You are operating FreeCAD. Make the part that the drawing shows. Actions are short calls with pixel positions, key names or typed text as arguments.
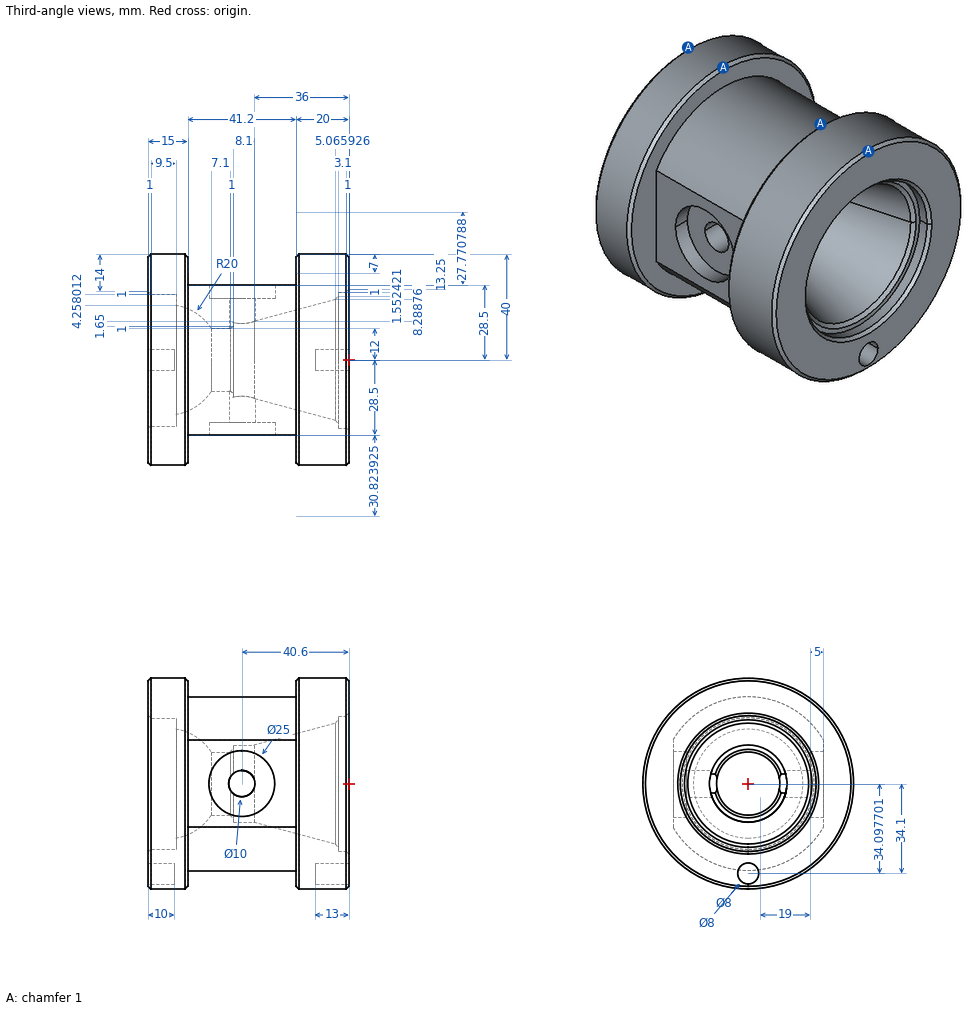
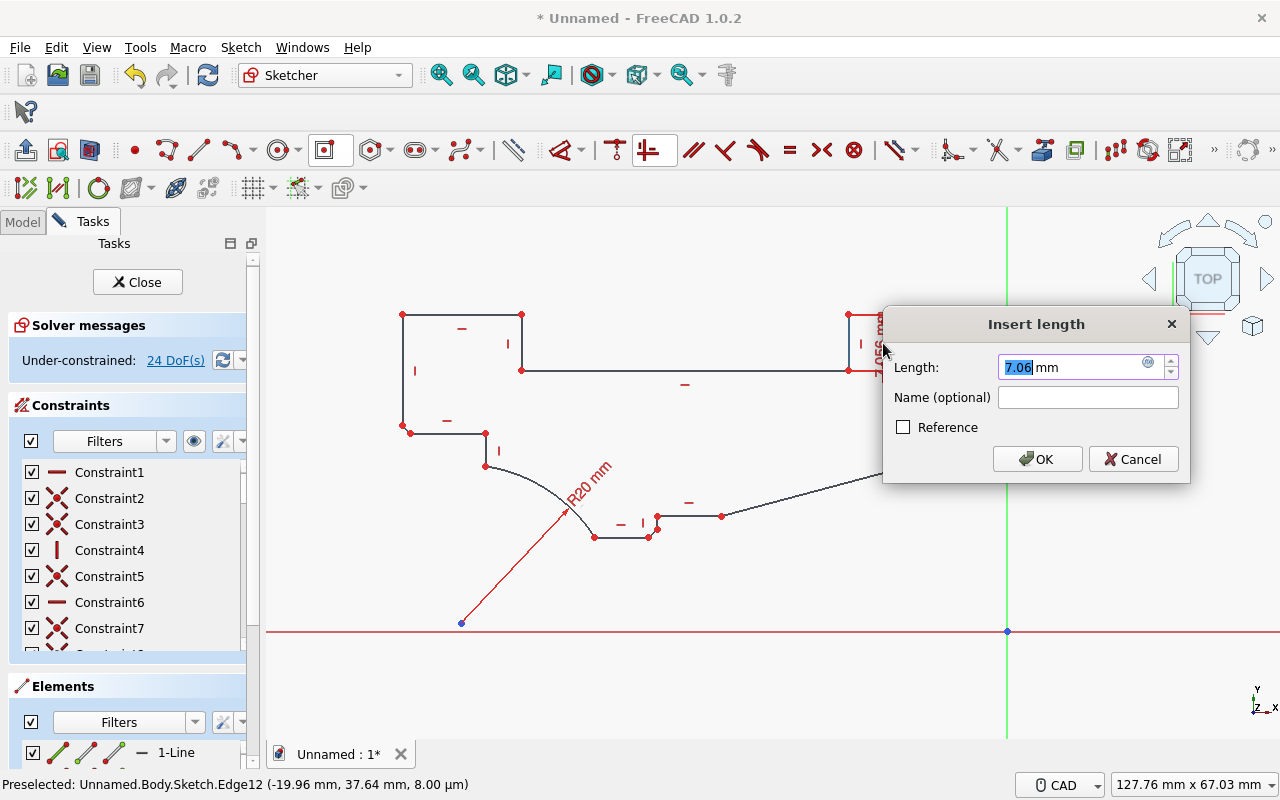
text(7)
key(Return)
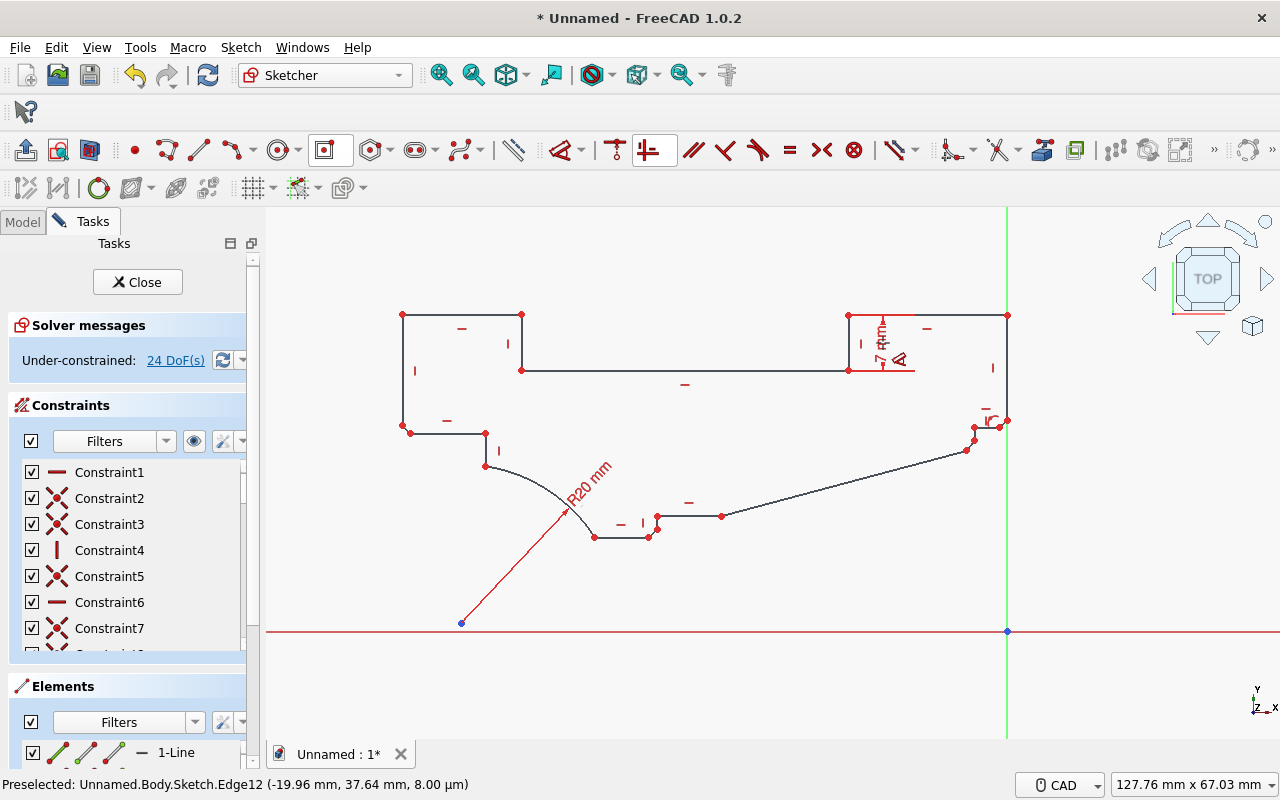
click(522, 354)
click(488, 343)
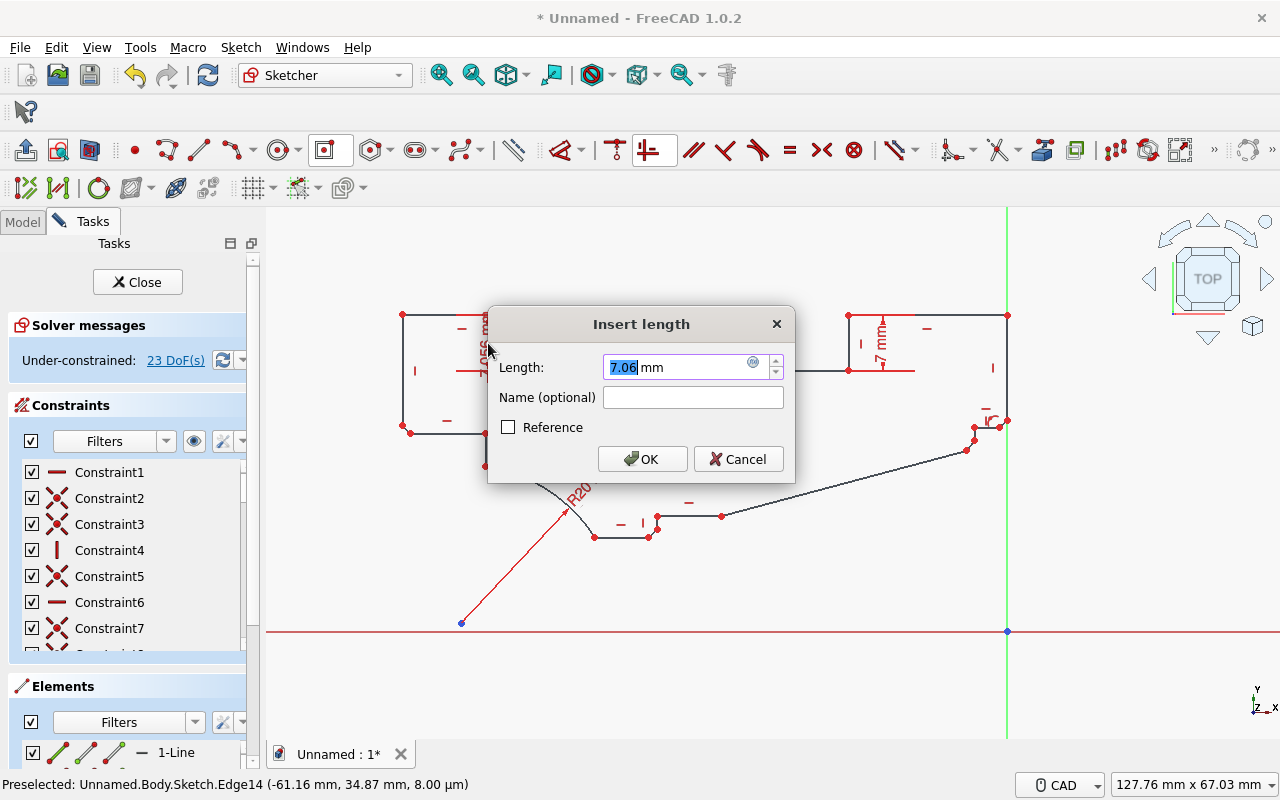
text(7)
key(Return)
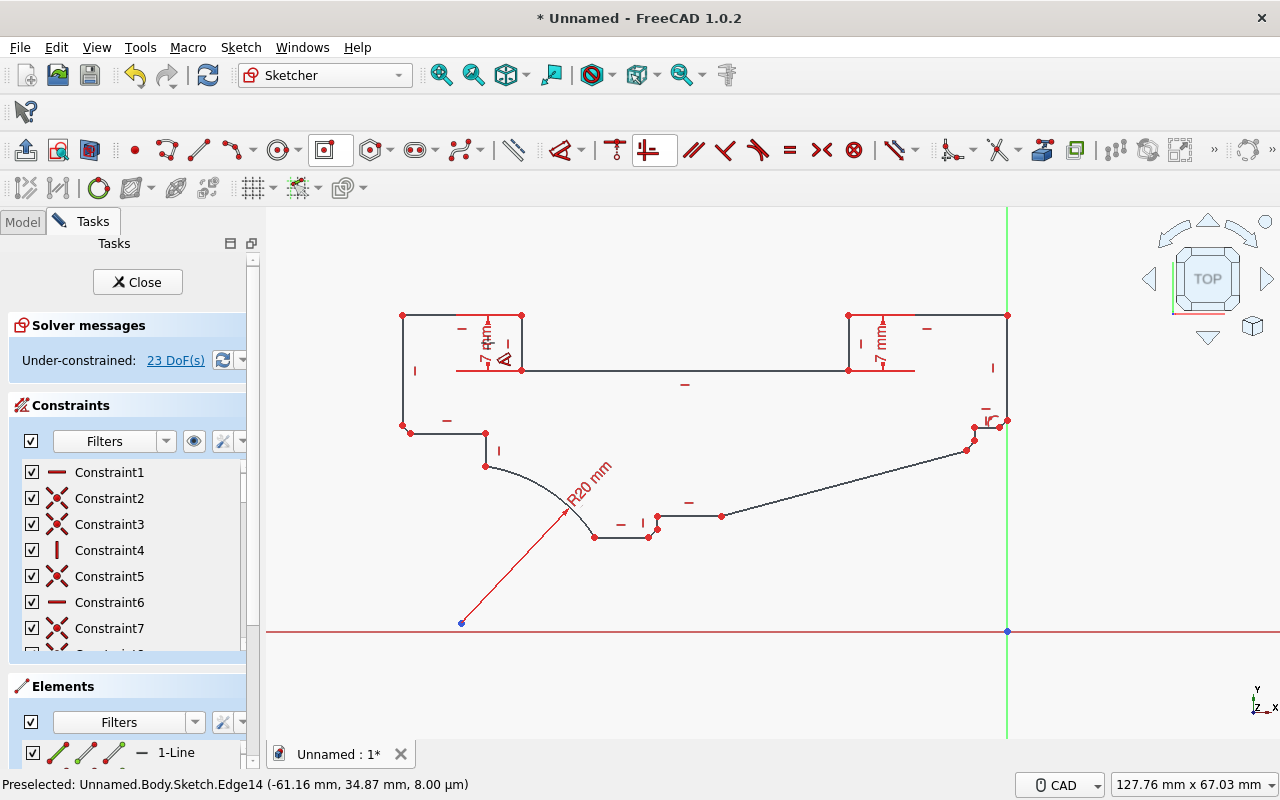
click(960, 315)
click(928, 281)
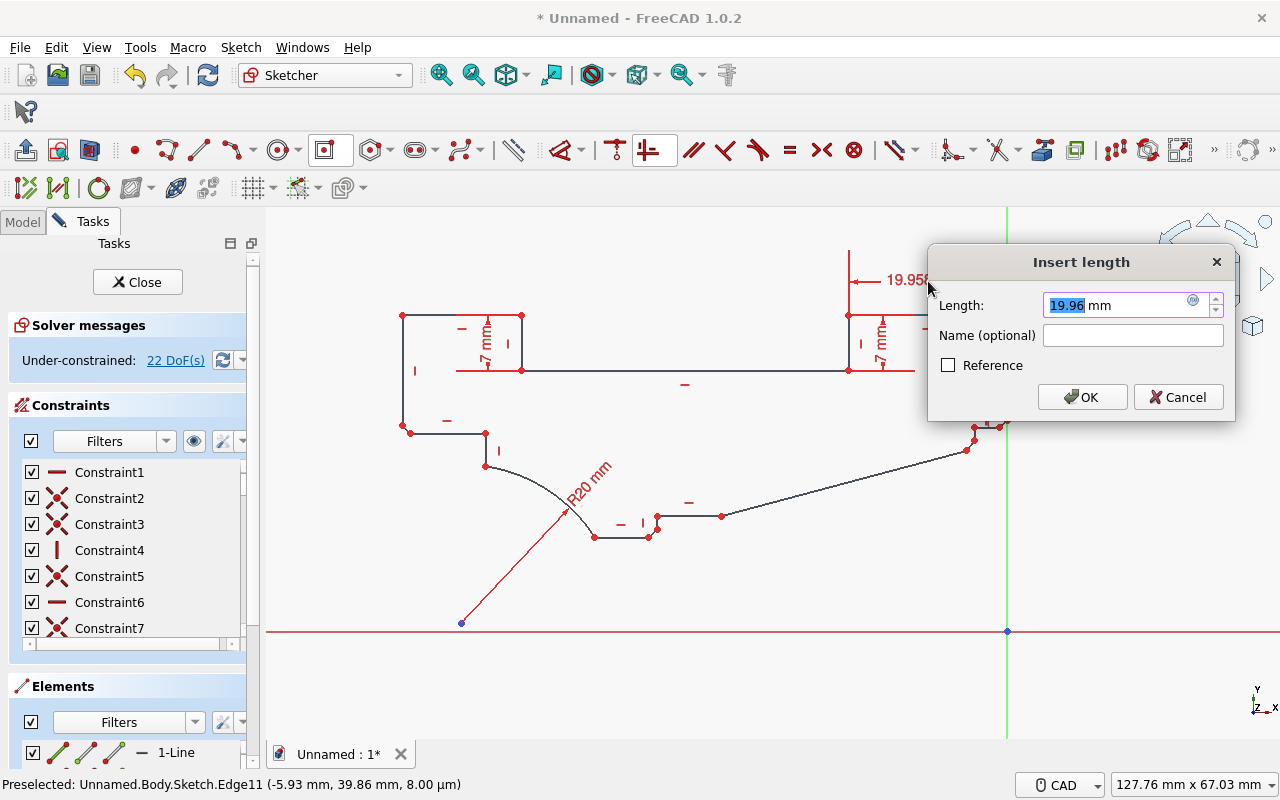
text(20)
key(Return)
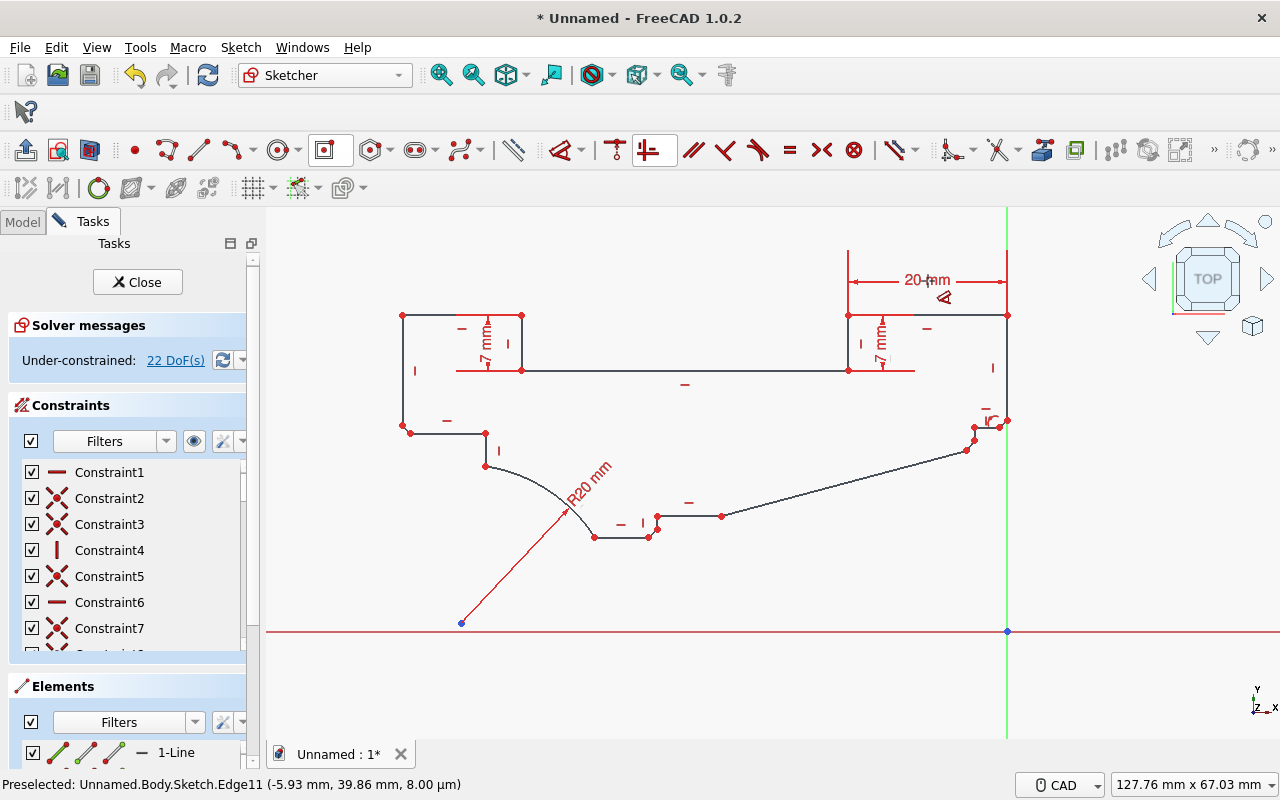
click(486, 315)
click(462, 281)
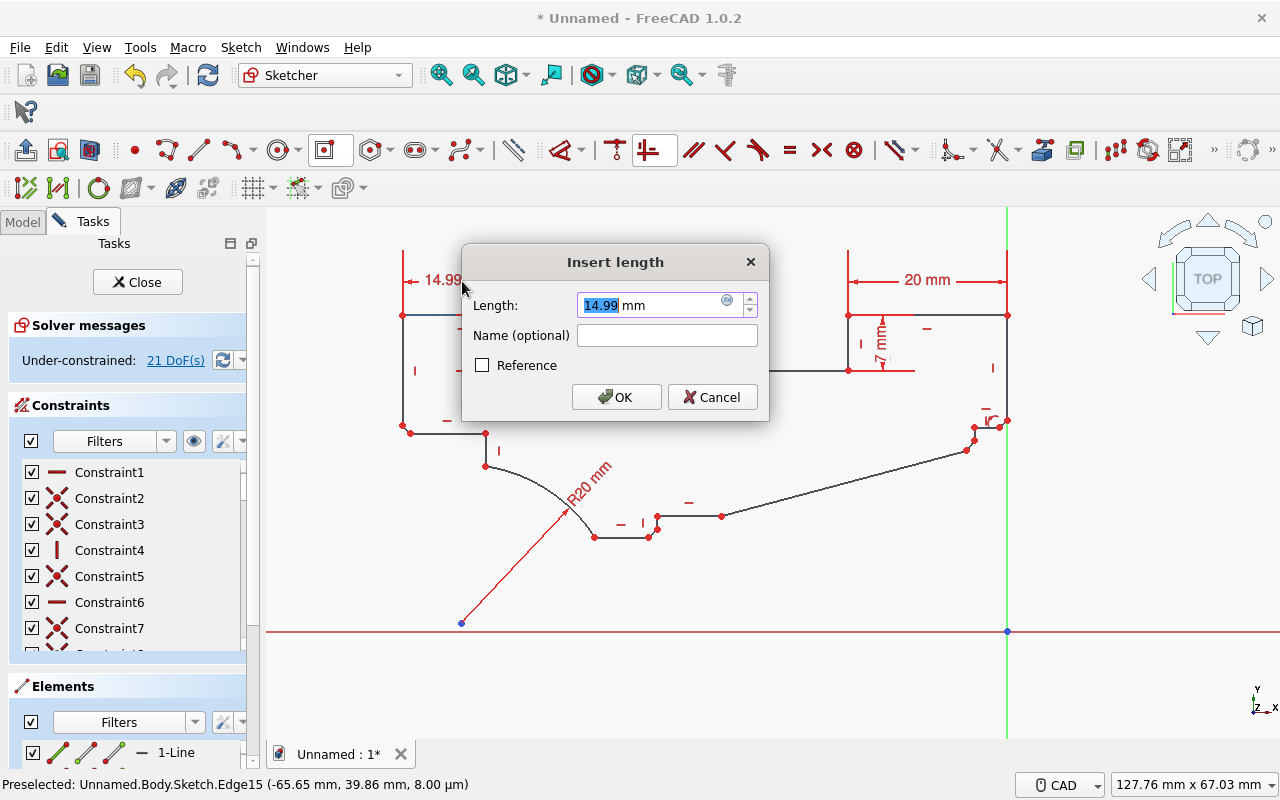
text(15)
key(Return)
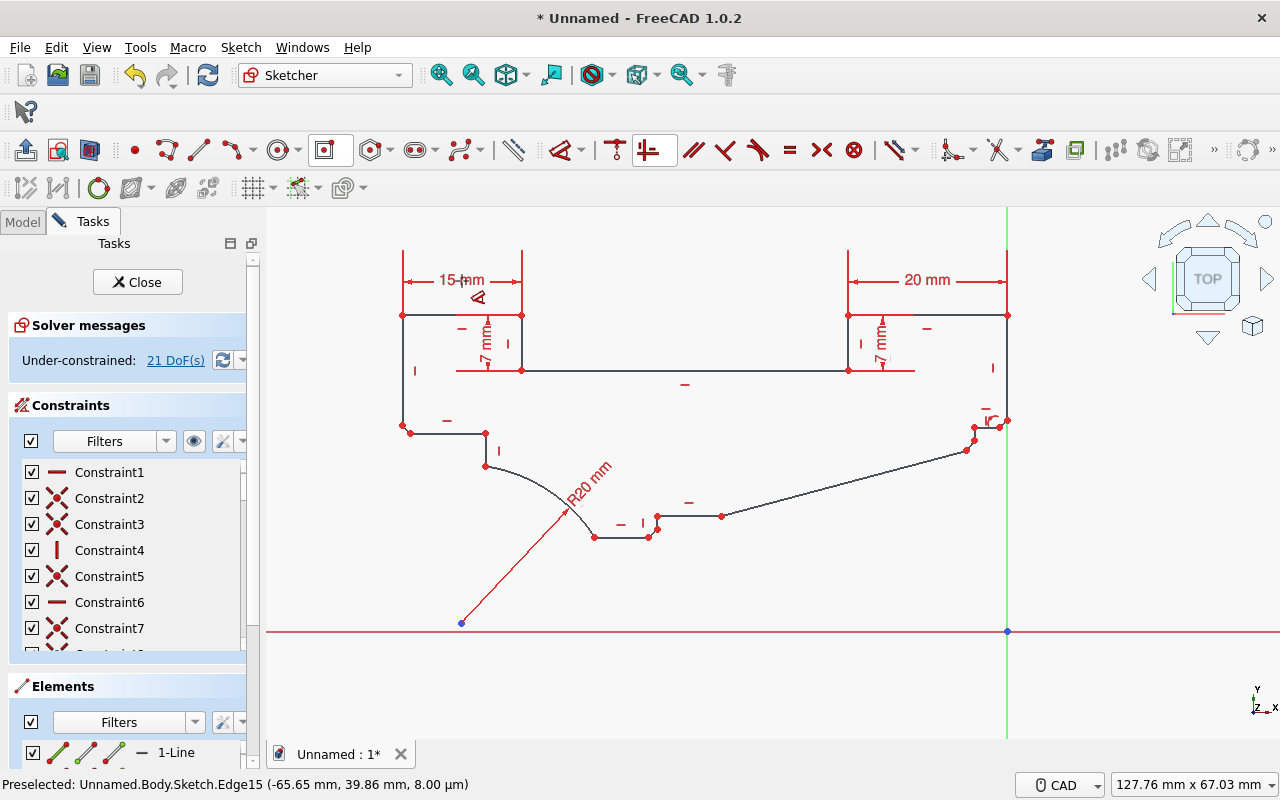
click(403, 349)
click(369, 371)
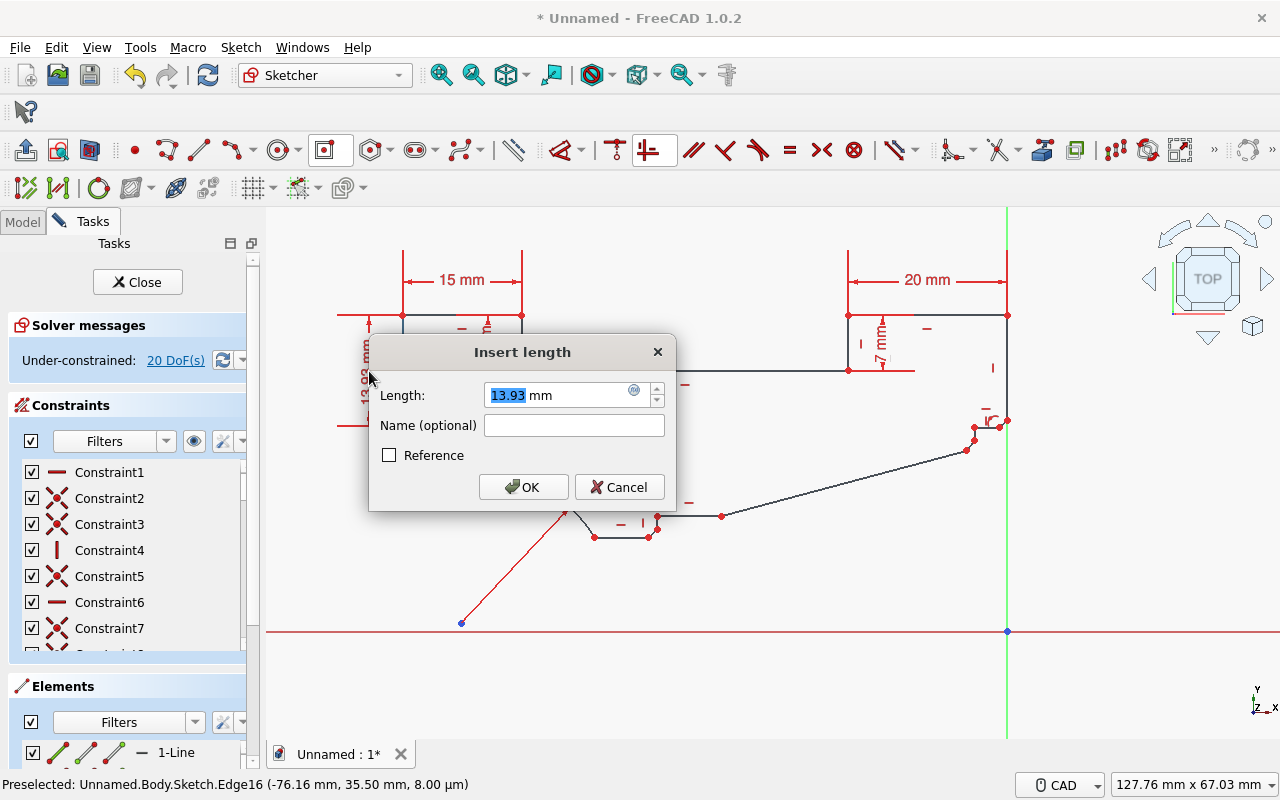
text(14)
key(Return)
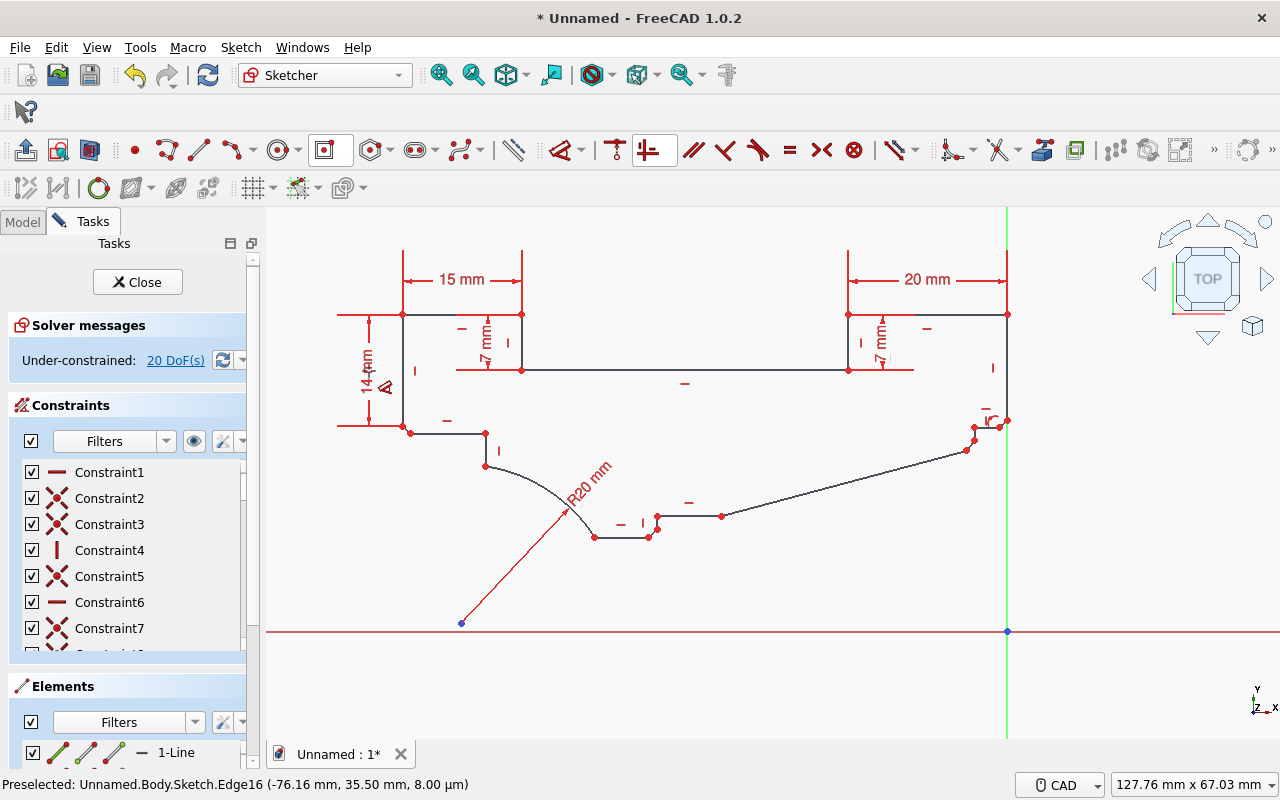
scroll(999, 428, up, 9)